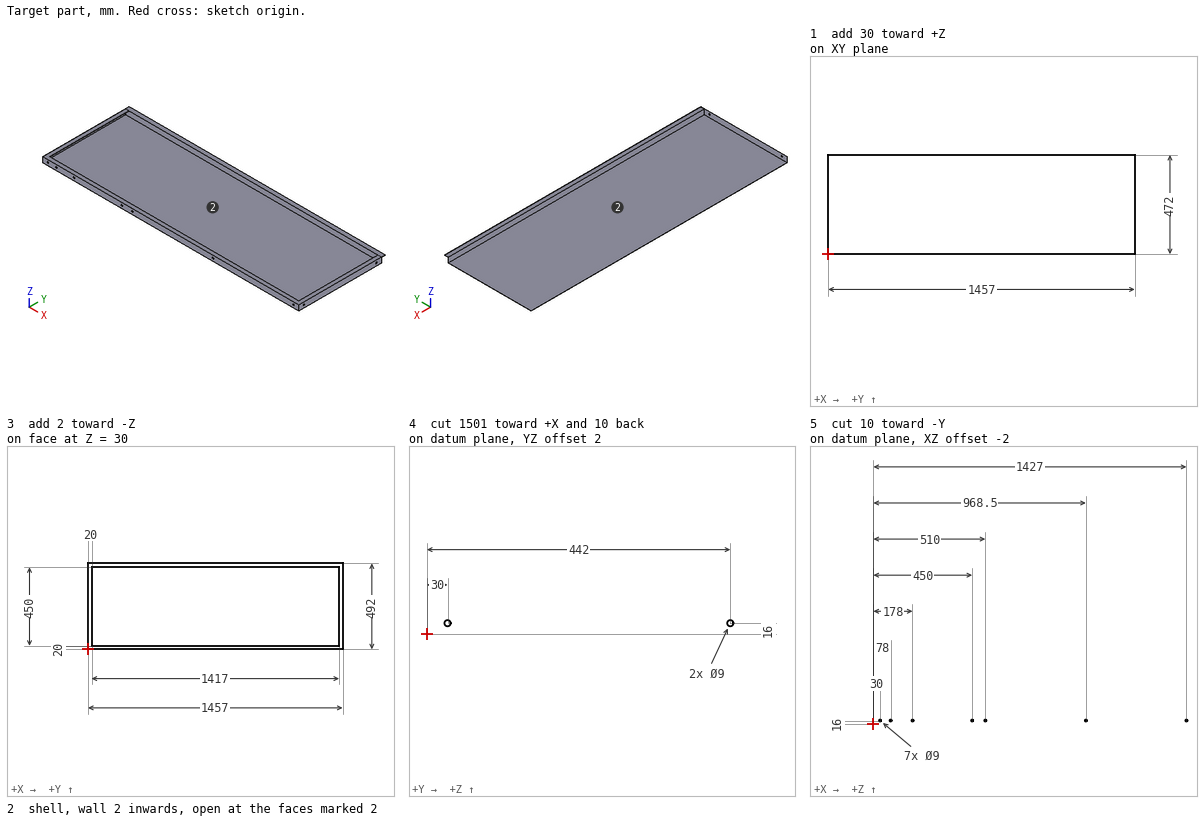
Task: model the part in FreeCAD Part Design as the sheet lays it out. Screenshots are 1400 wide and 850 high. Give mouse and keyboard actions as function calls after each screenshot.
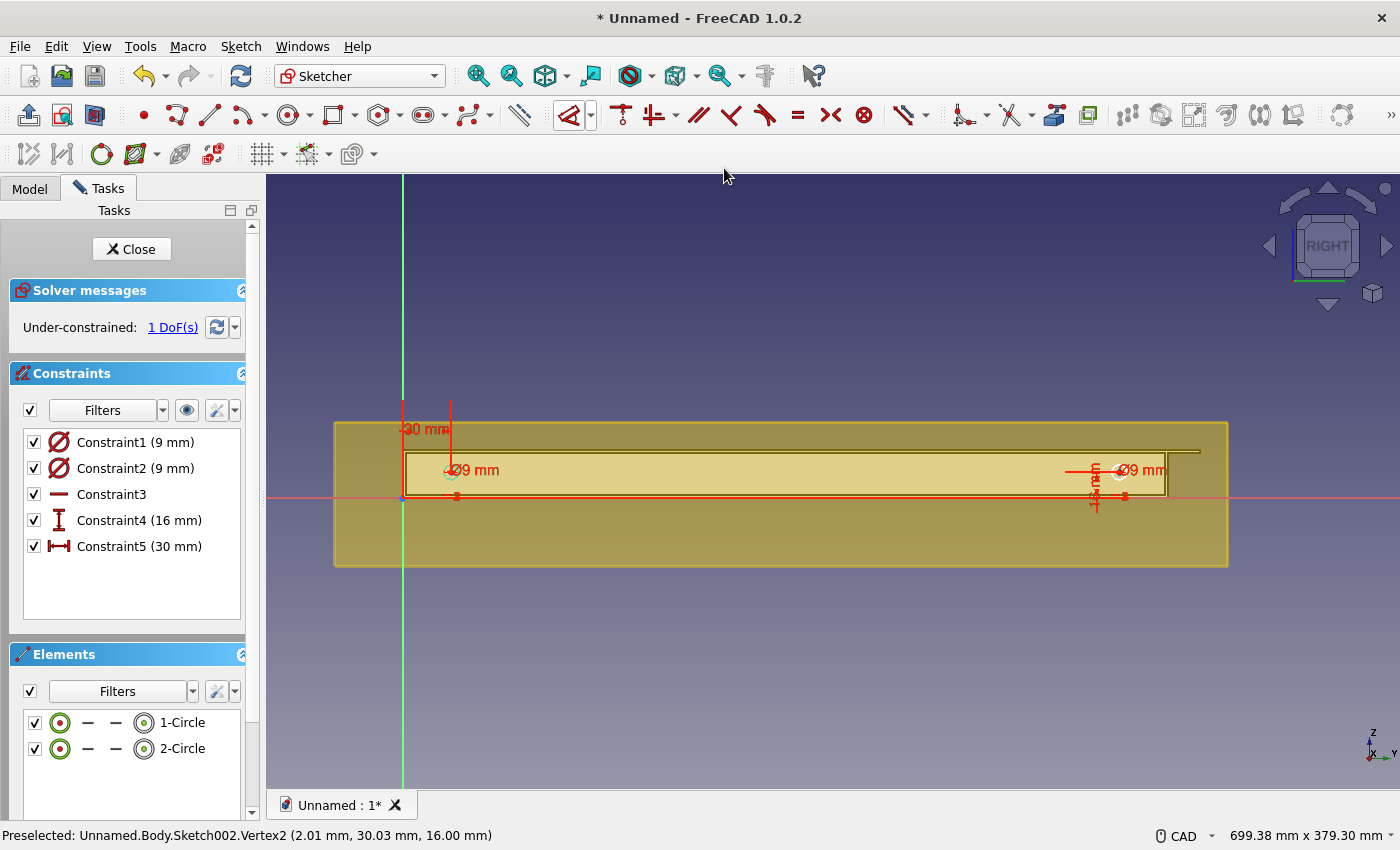
click(1119, 472)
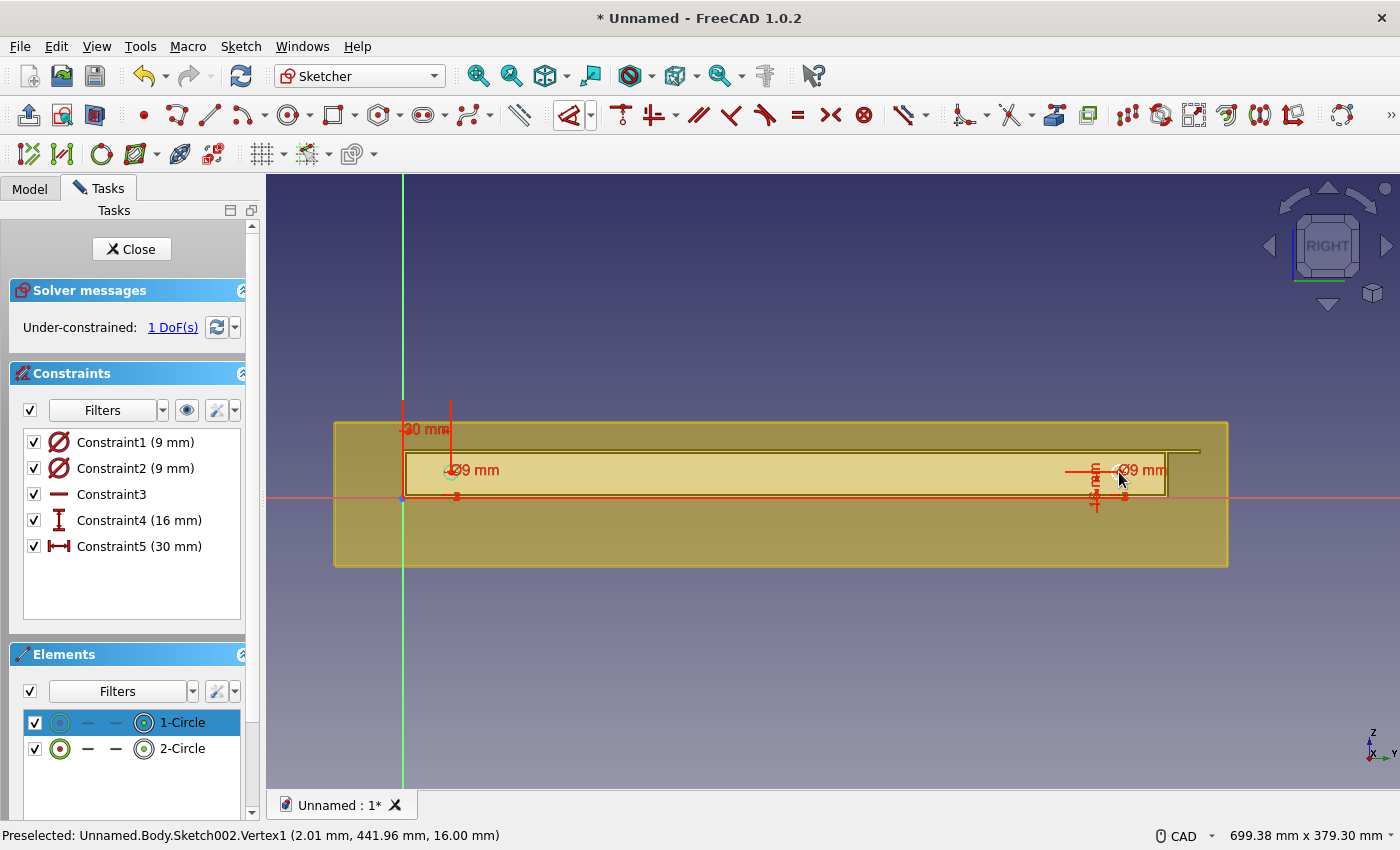
key(l)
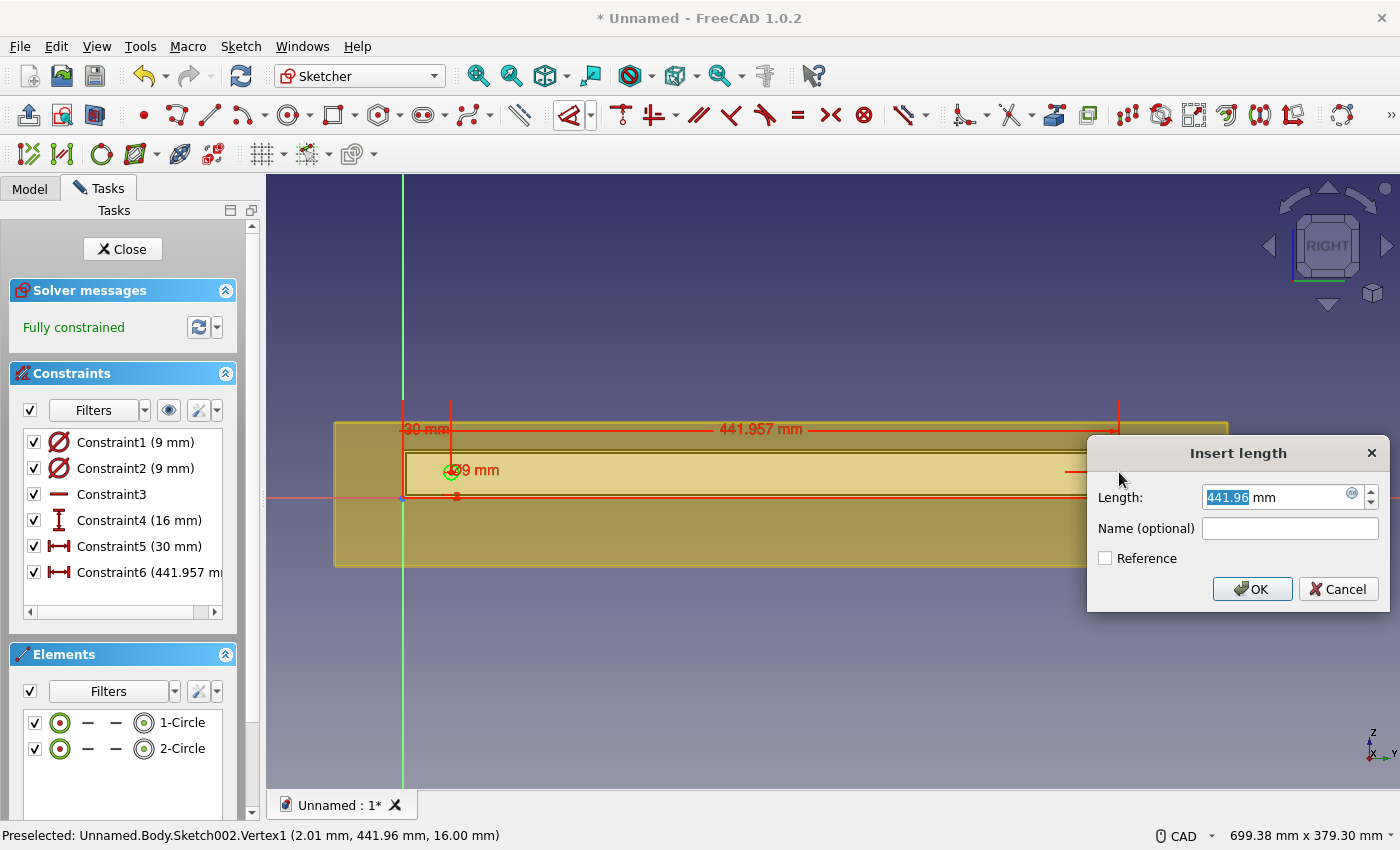
text(442)
key(Return)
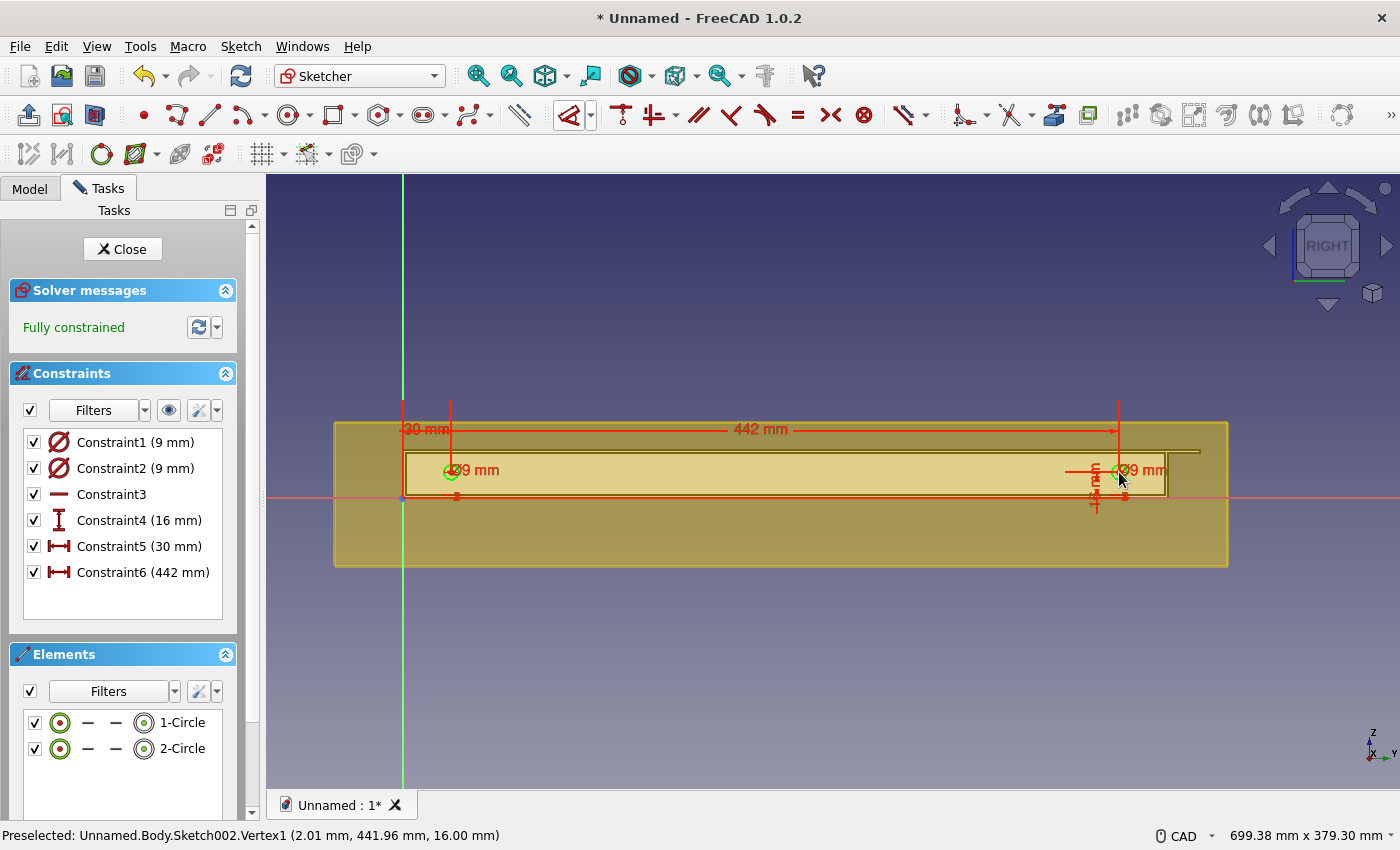
click(123, 249)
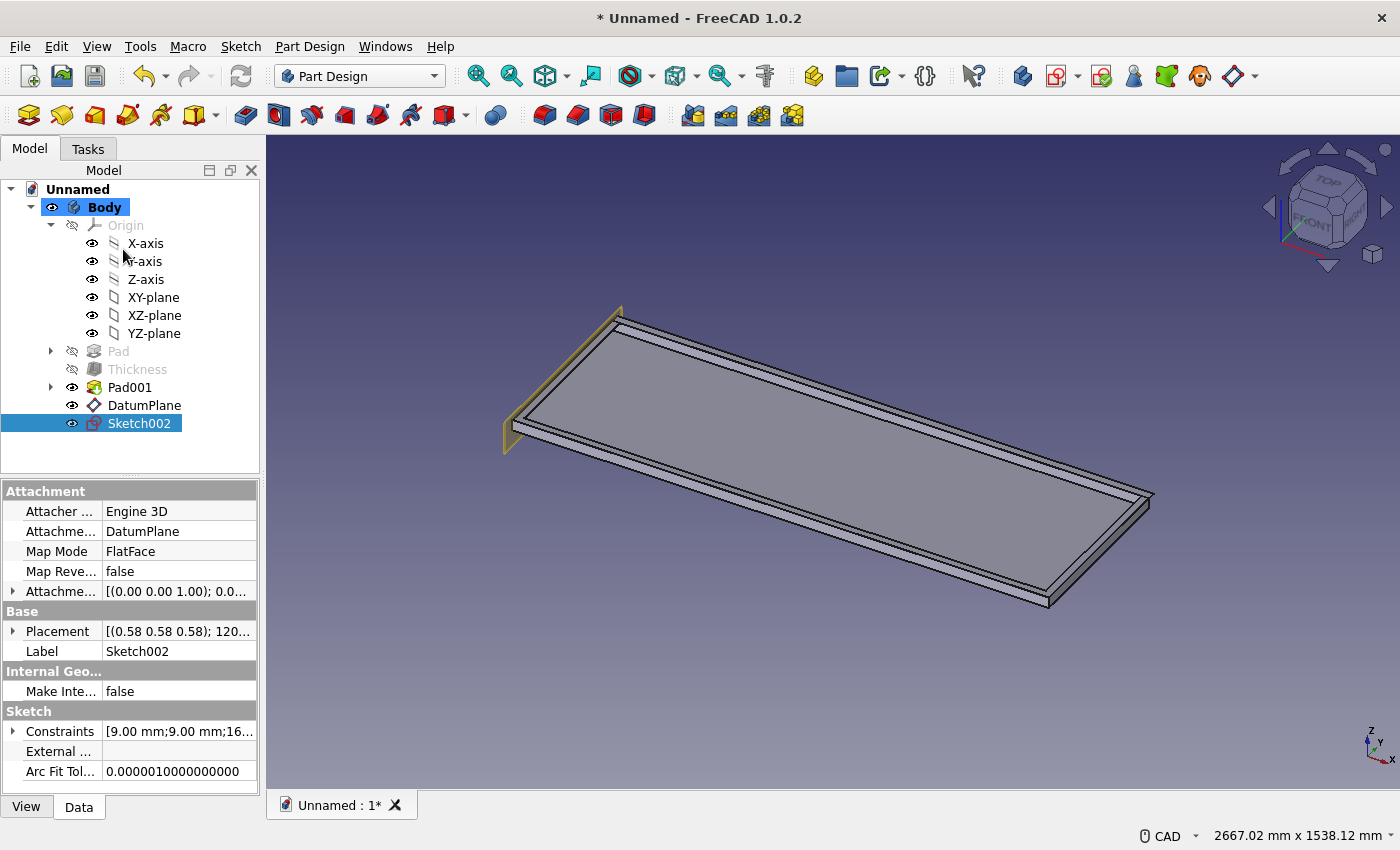
click(246, 116)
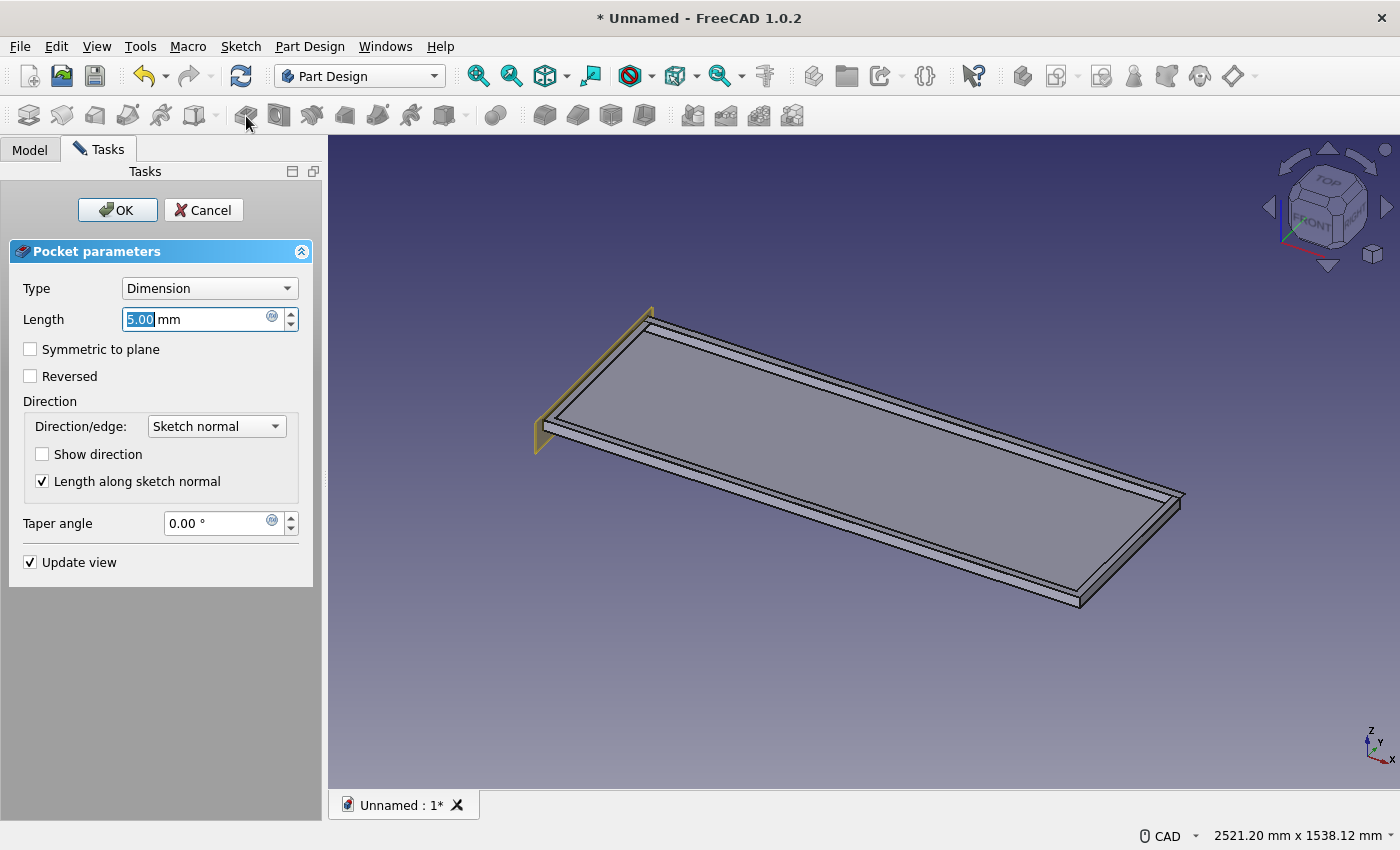
click(210, 288)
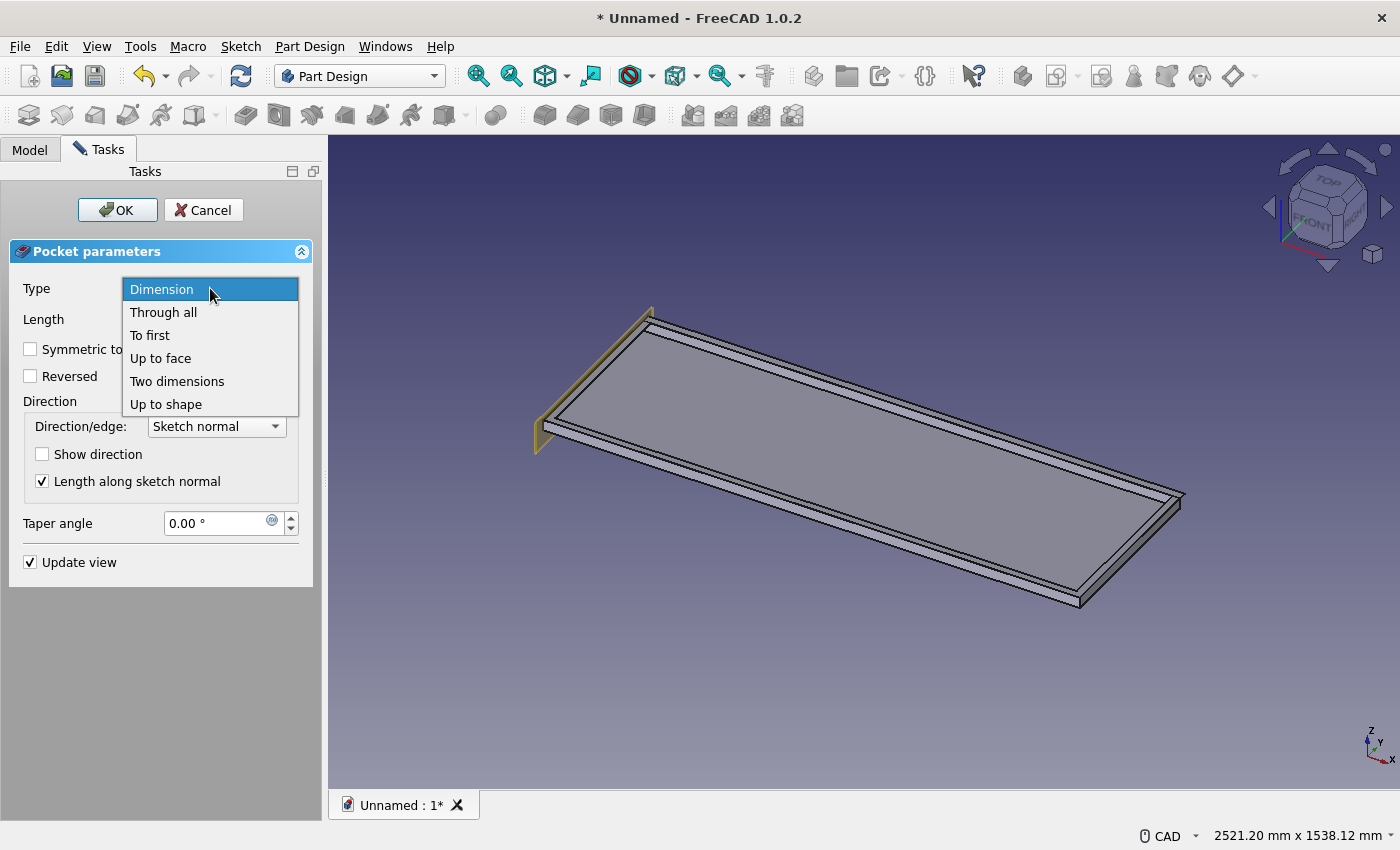
click(208, 382)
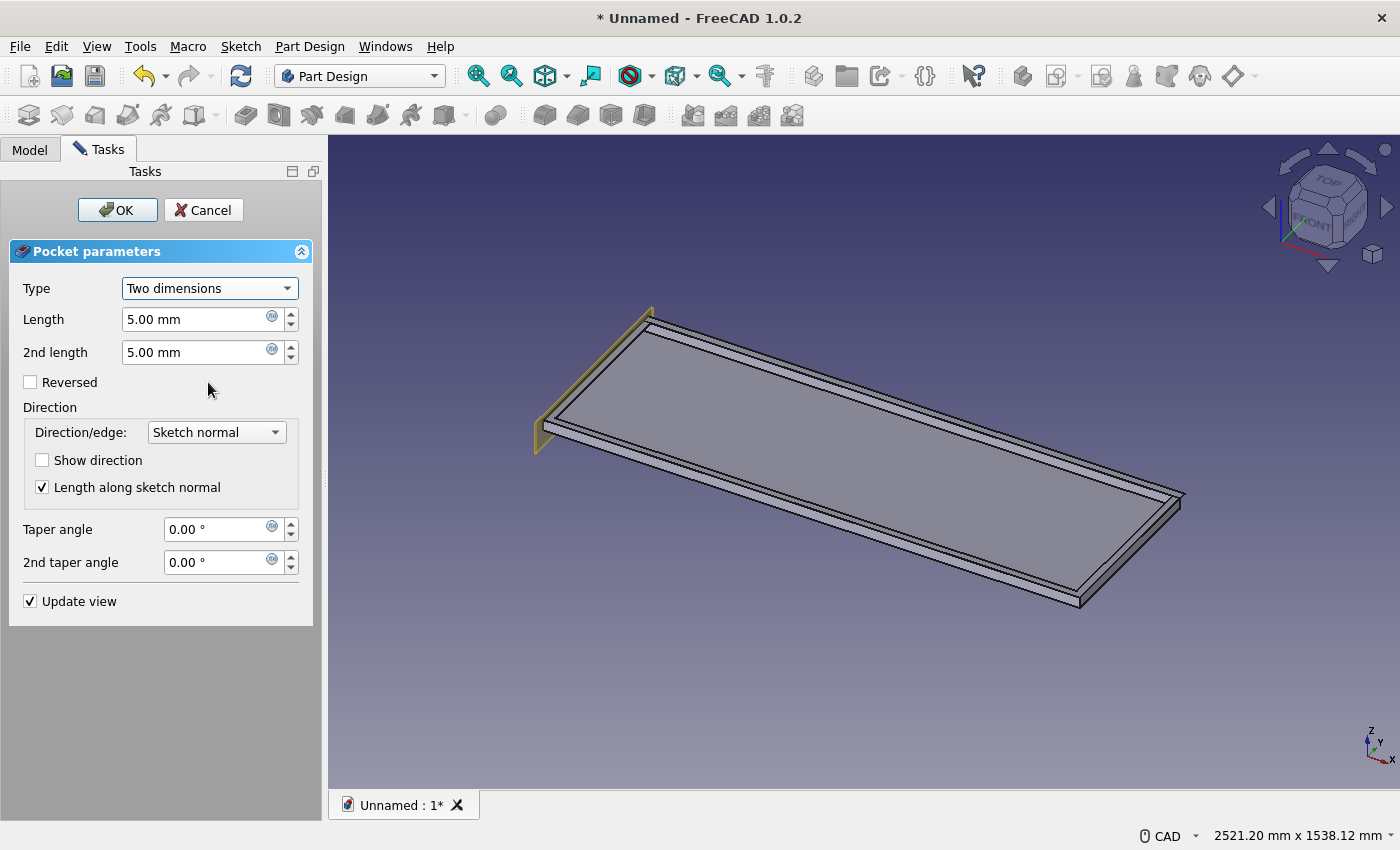
triple_click(204, 320)